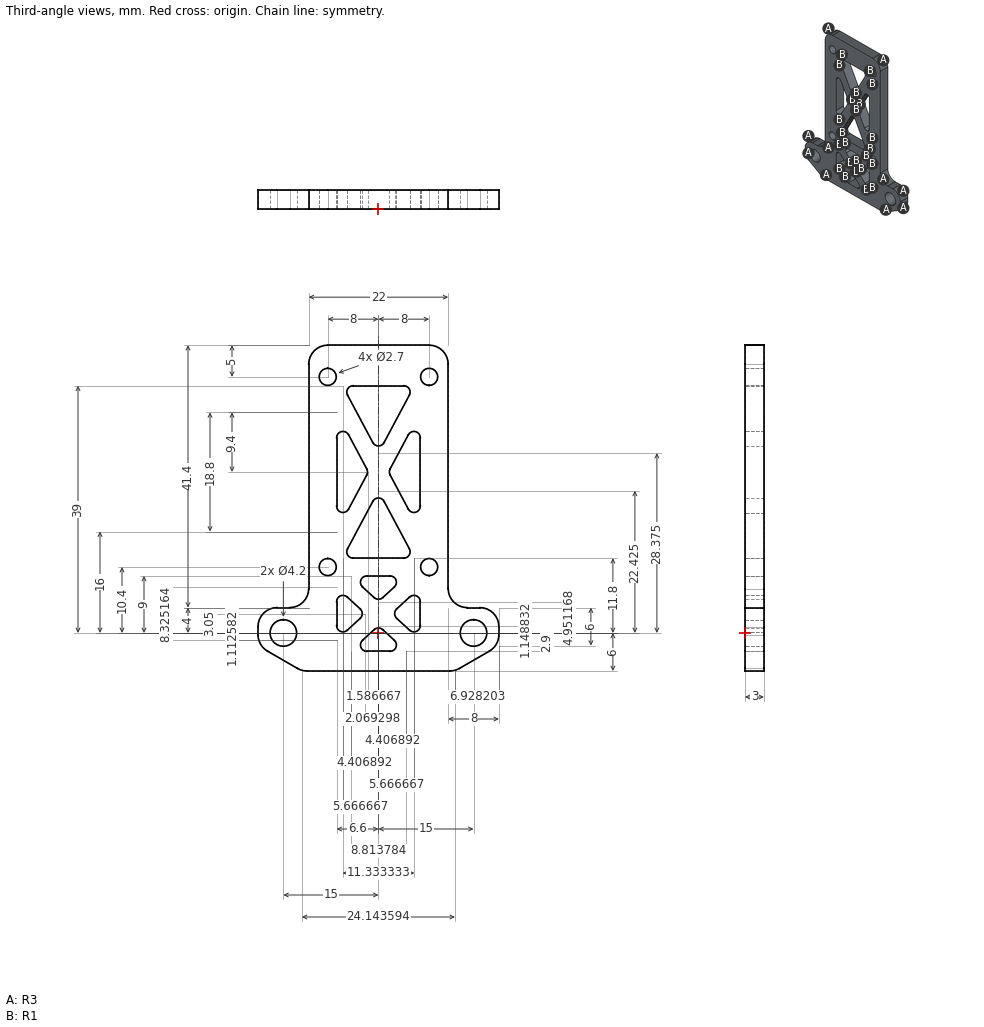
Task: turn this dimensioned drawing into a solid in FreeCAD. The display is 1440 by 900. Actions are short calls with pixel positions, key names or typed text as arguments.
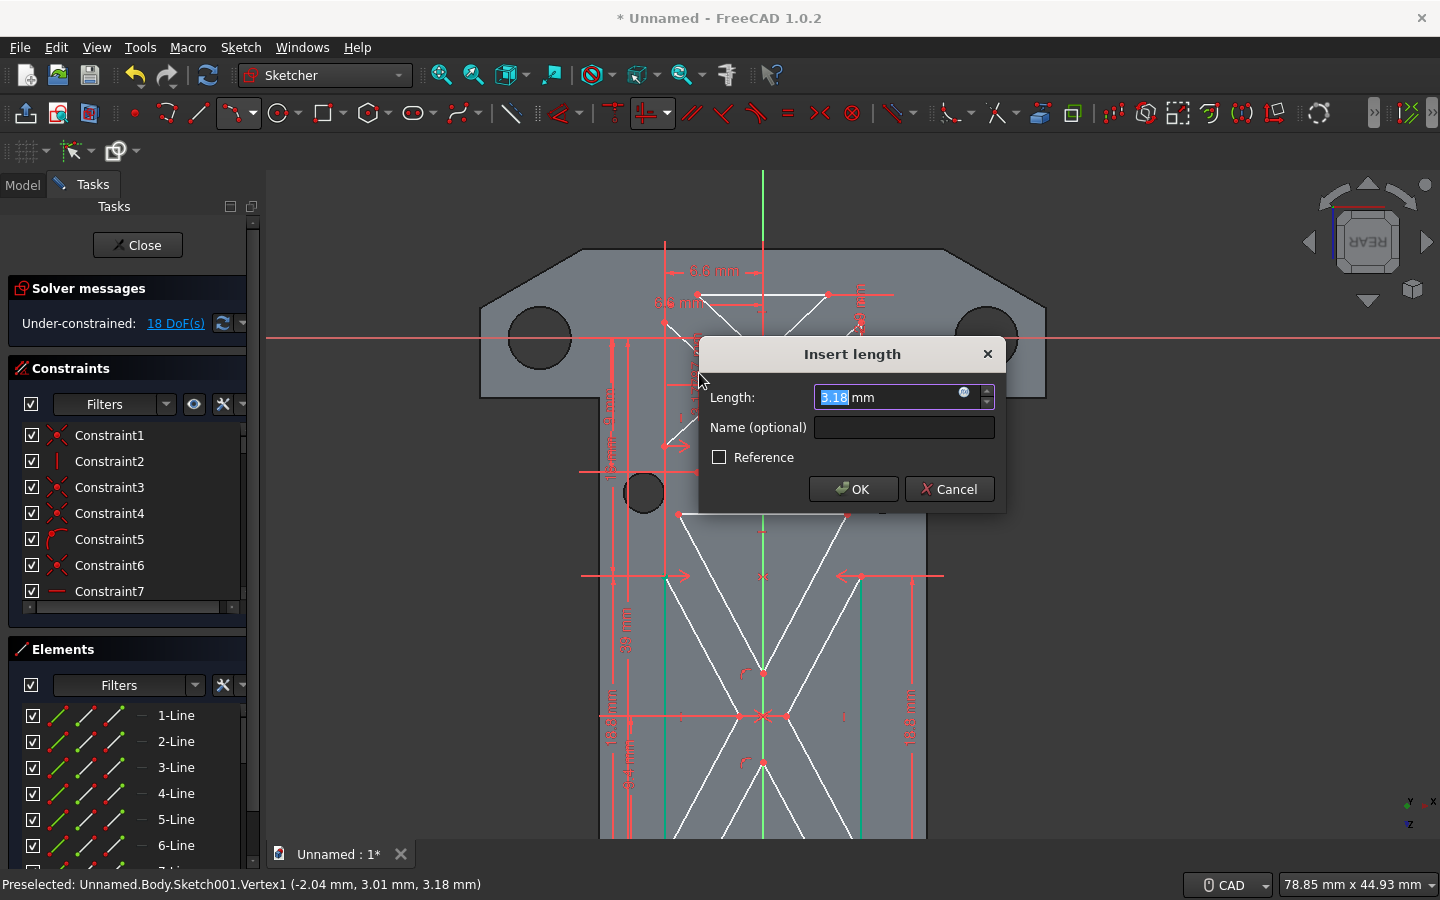
text(3.05)
key(Return)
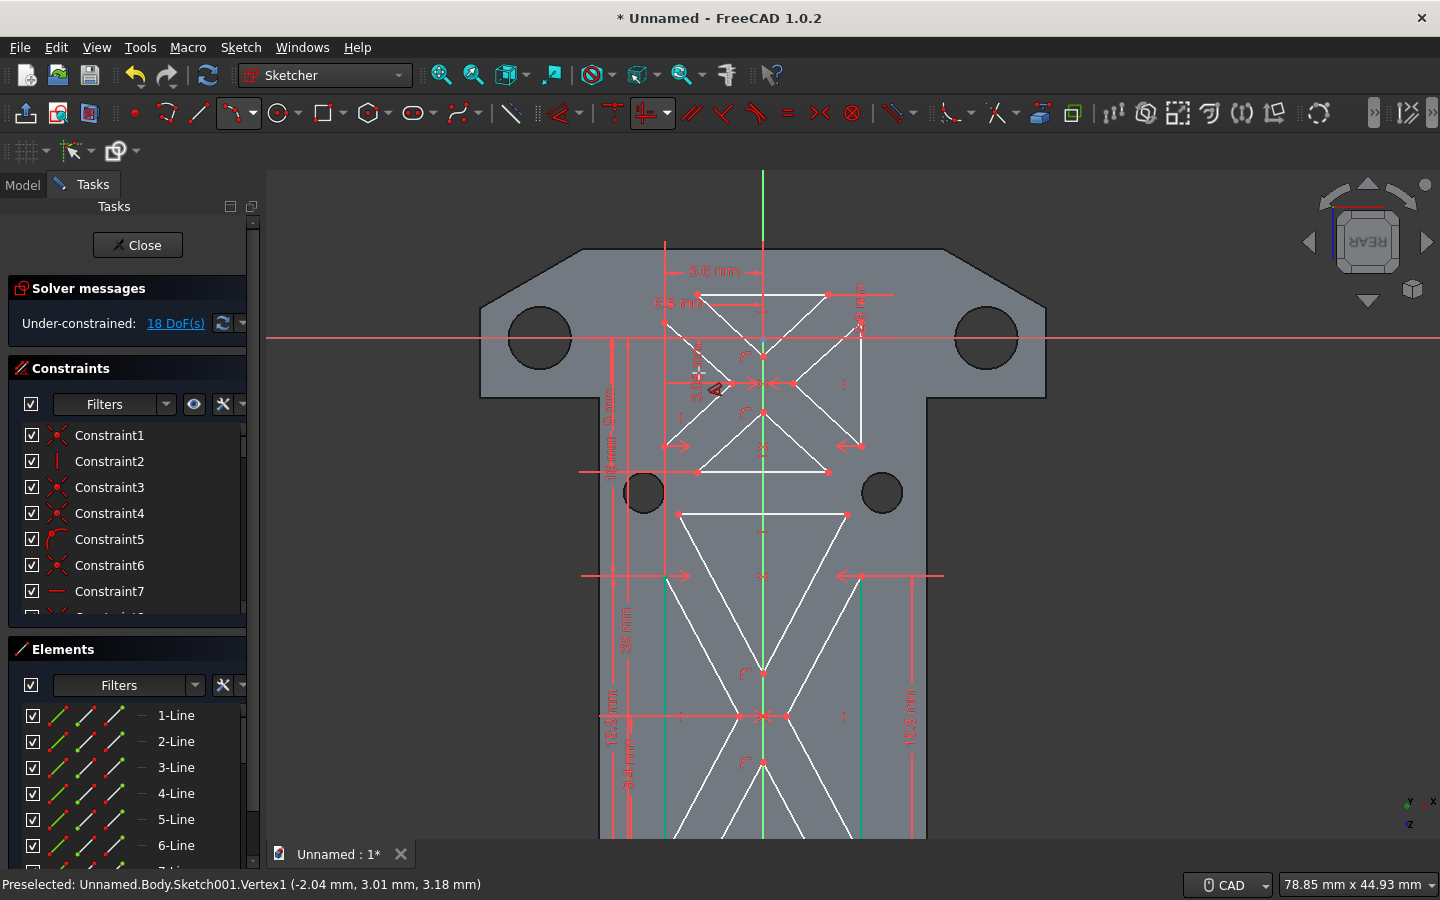
click(847, 514)
click(881, 426)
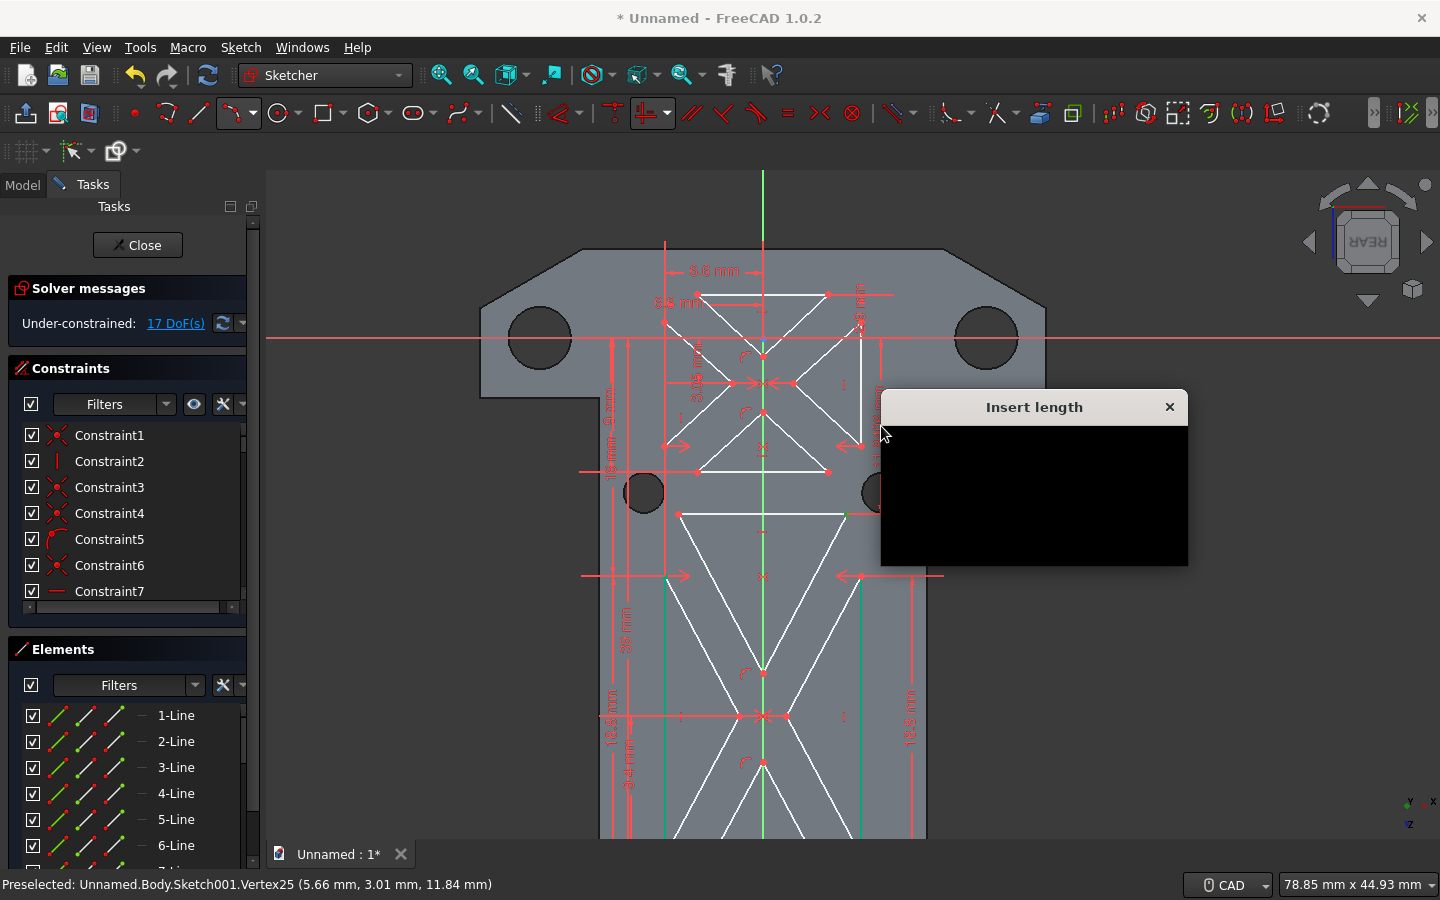
text(11.8)
key(Return)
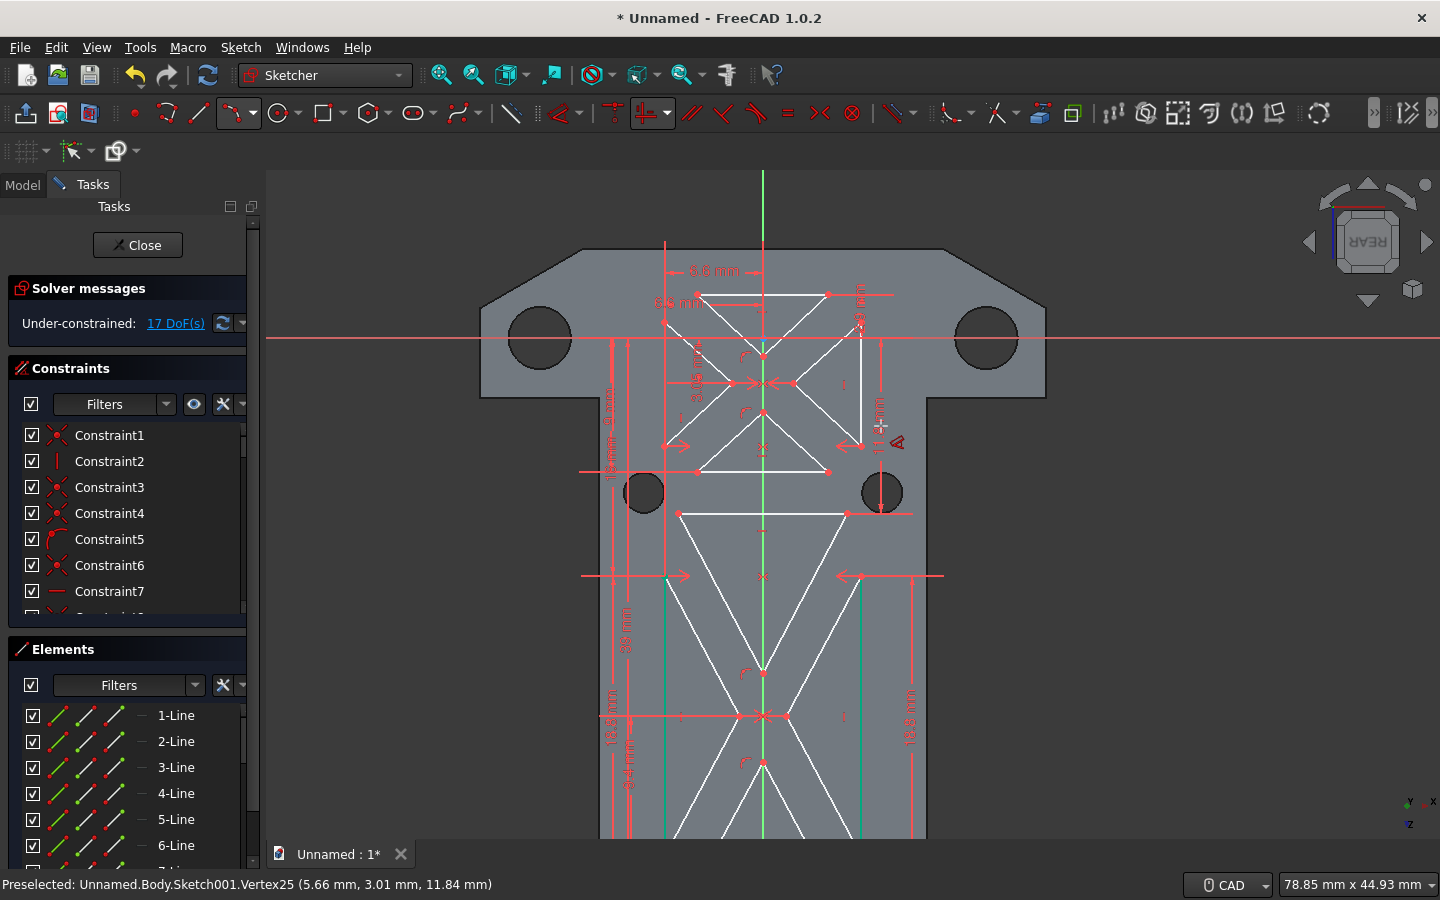
click(763, 673)
click(821, 388)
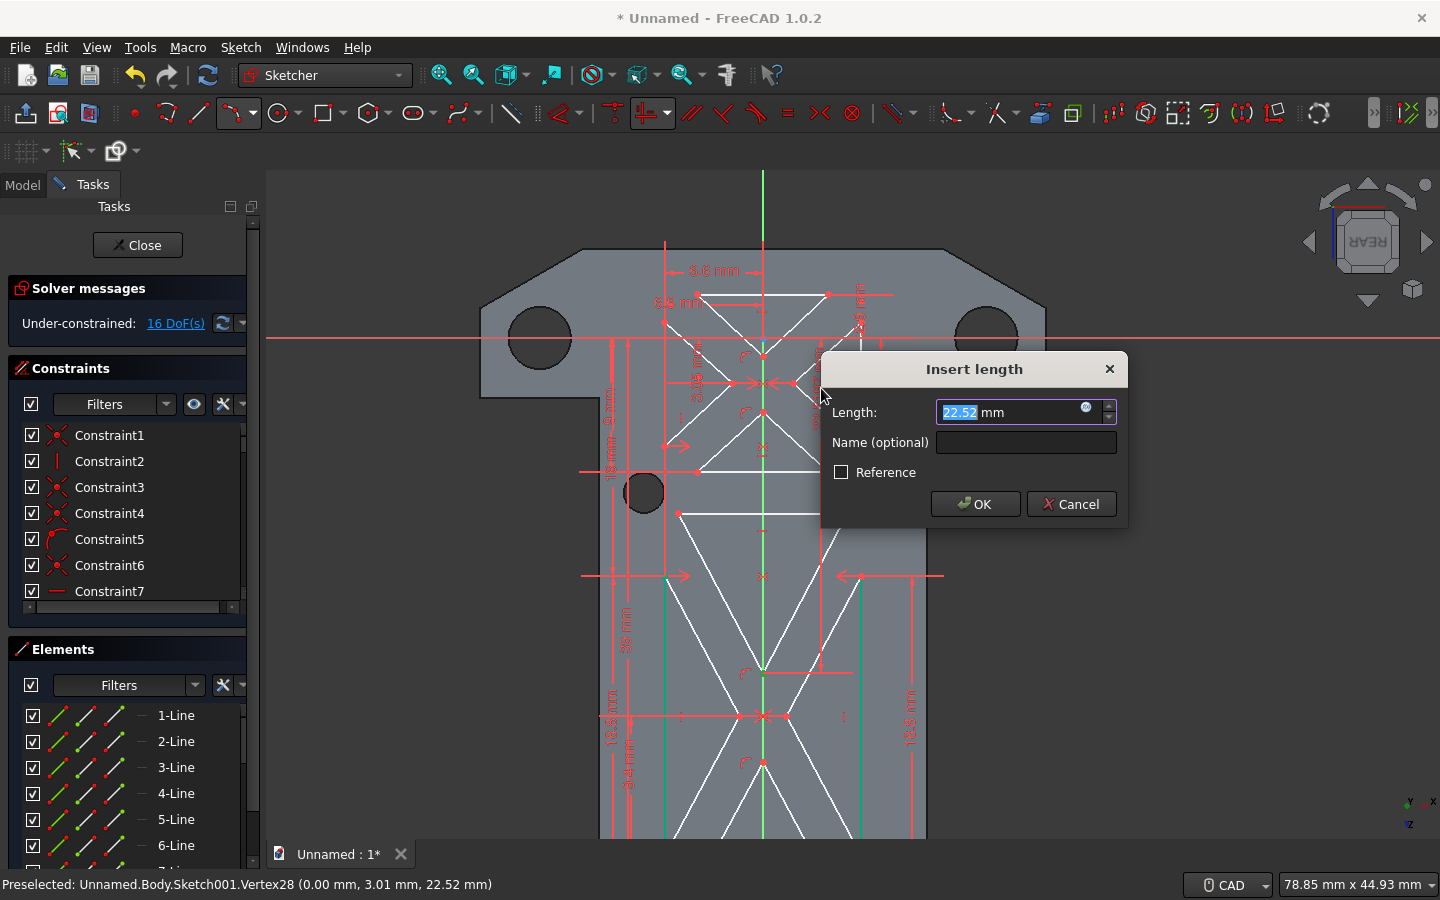
text(22.425)
key(Return)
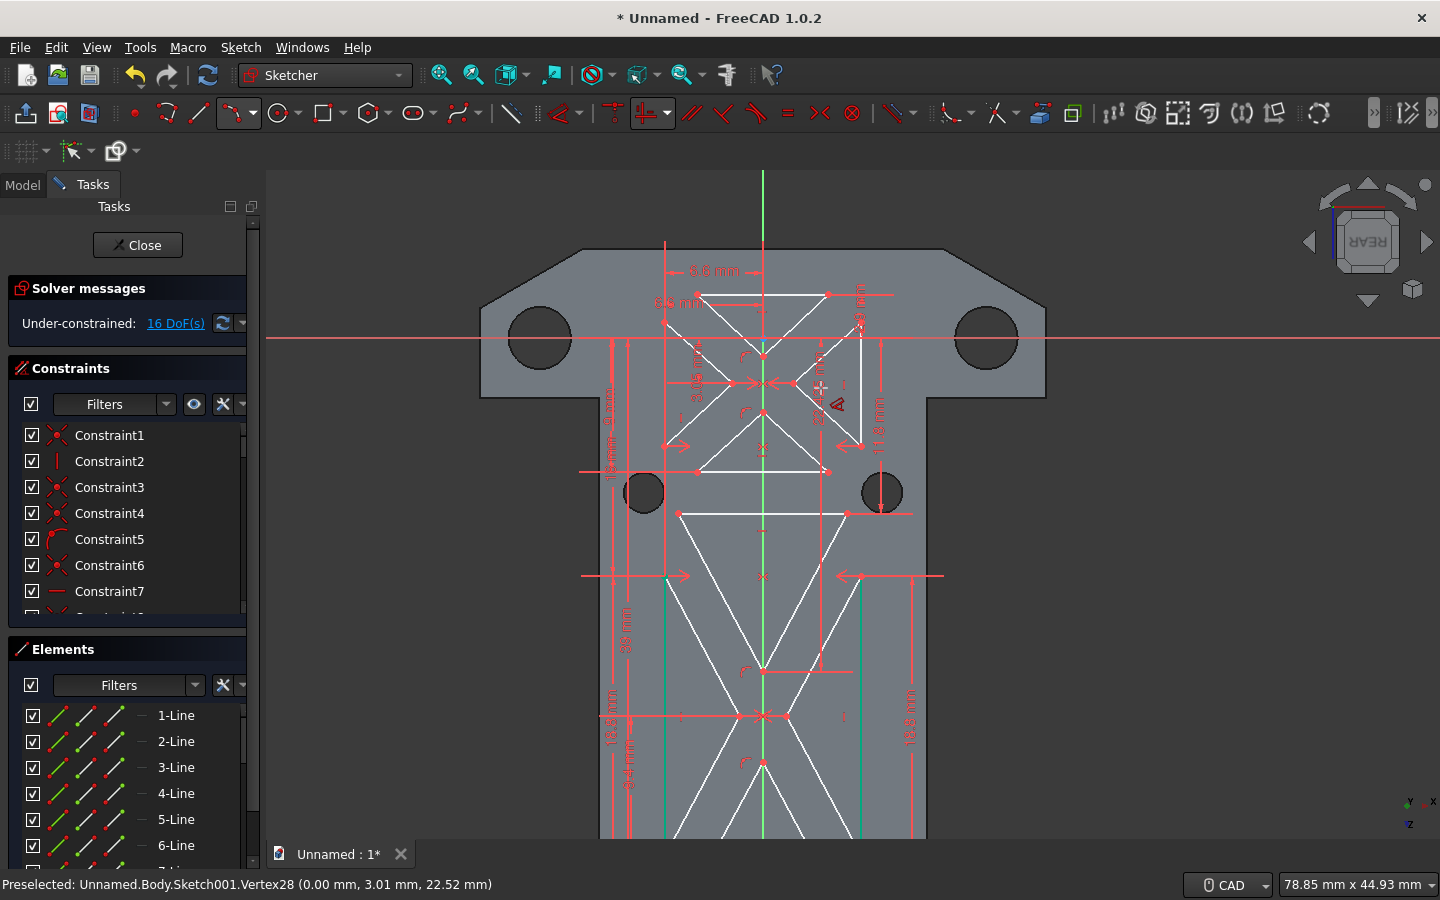
click(763, 762)
click(797, 550)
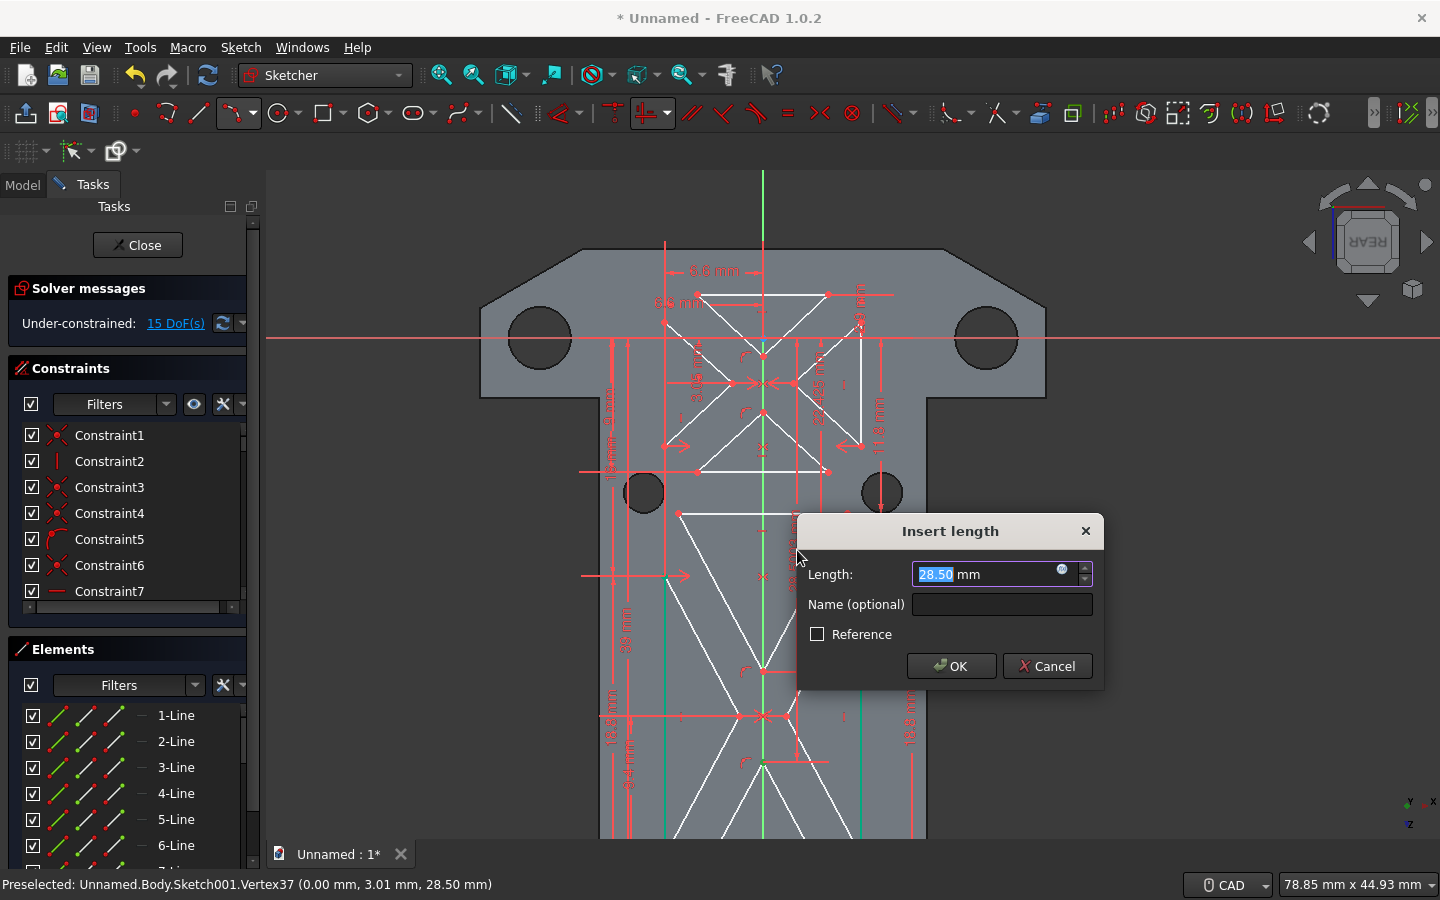
text(28.375)
key(Return)